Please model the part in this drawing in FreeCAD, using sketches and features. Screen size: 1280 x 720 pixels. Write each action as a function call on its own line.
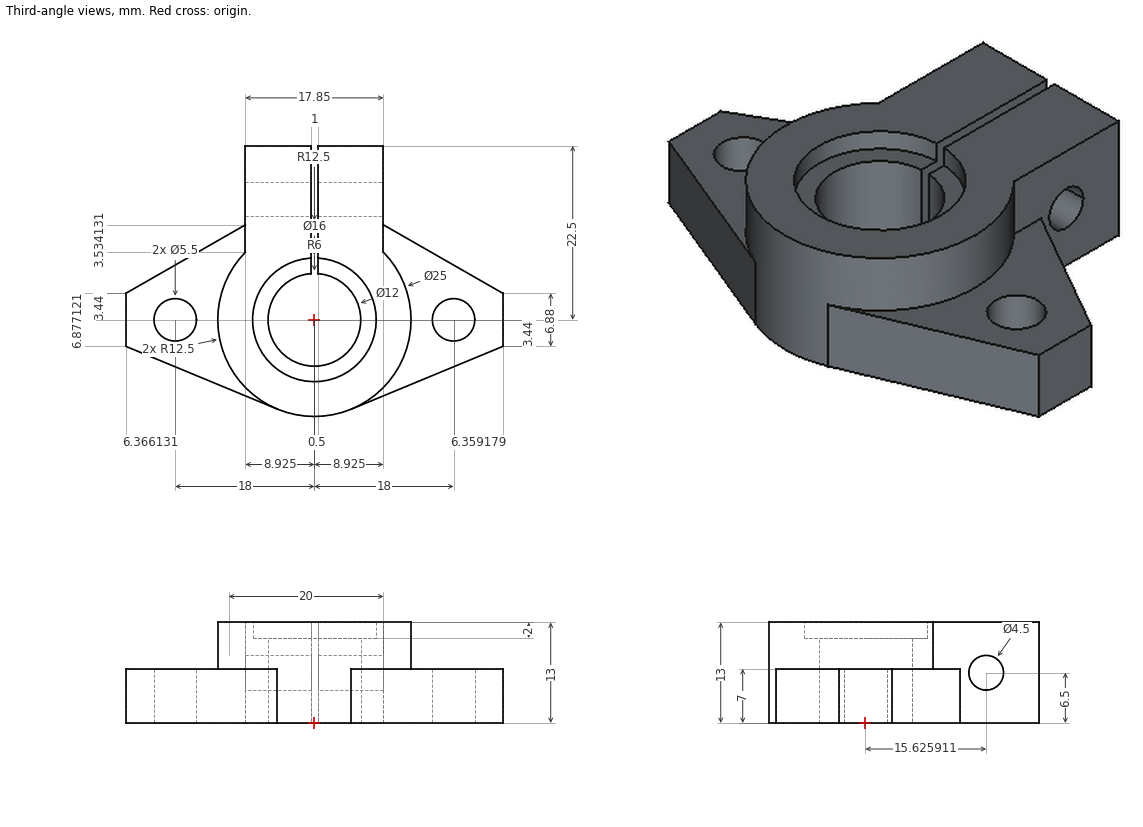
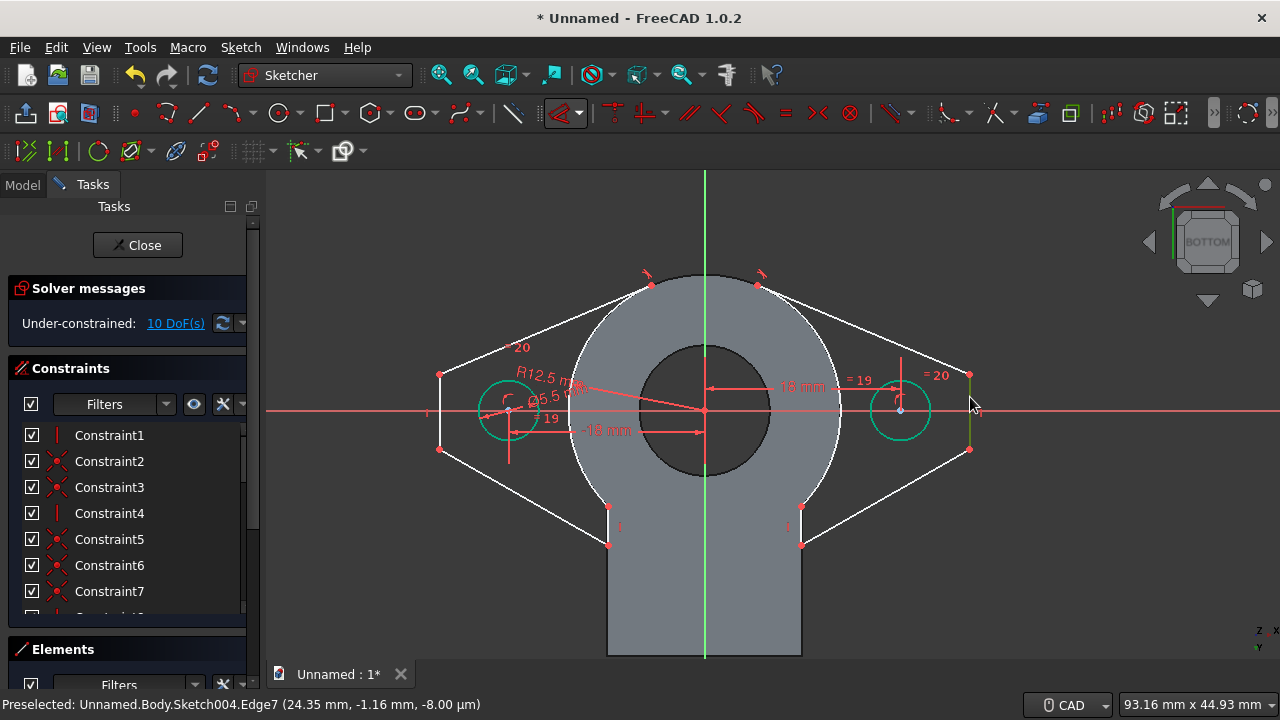
click(582, 114)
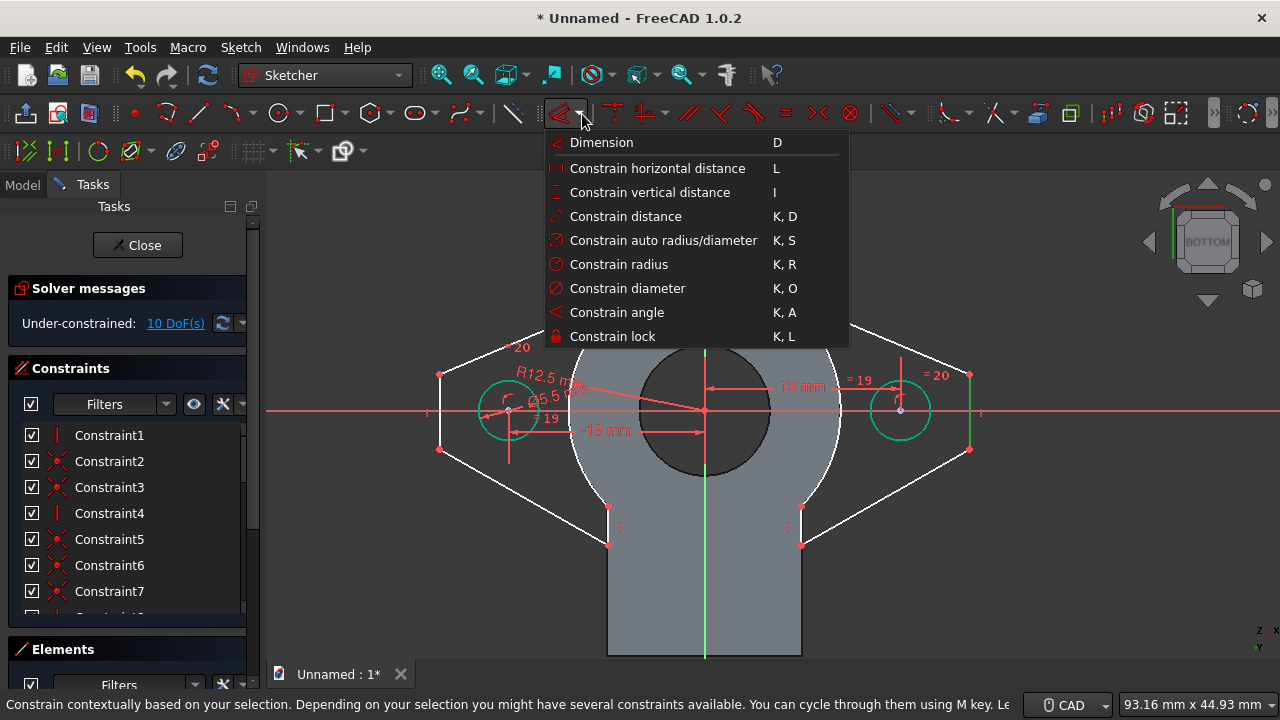
click(697, 192)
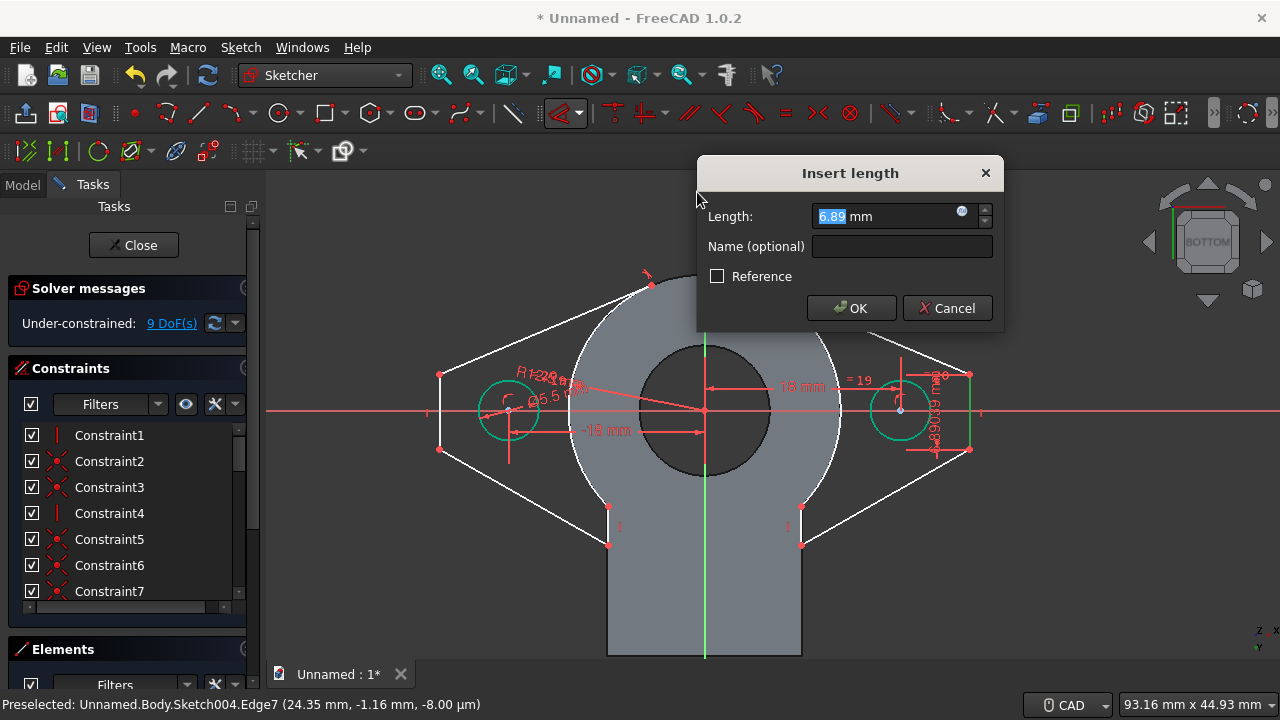
text(6.88)
key(Return)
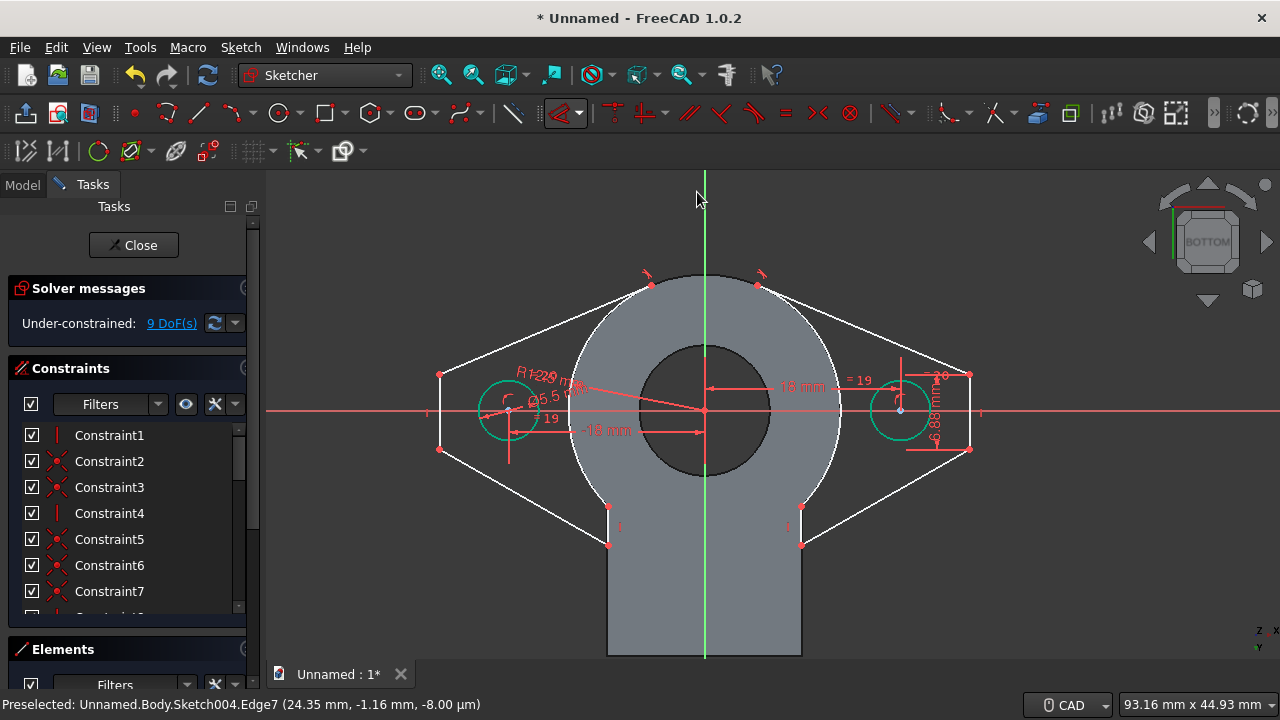
click(440, 450)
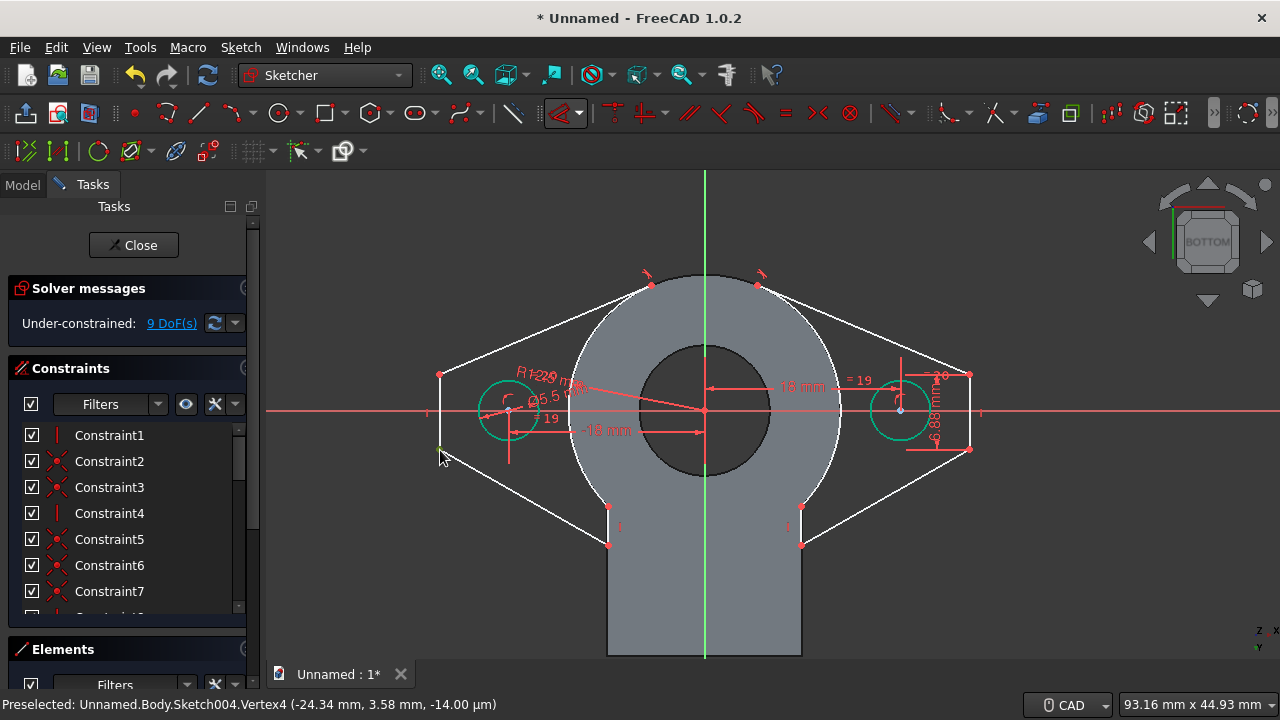
key(i)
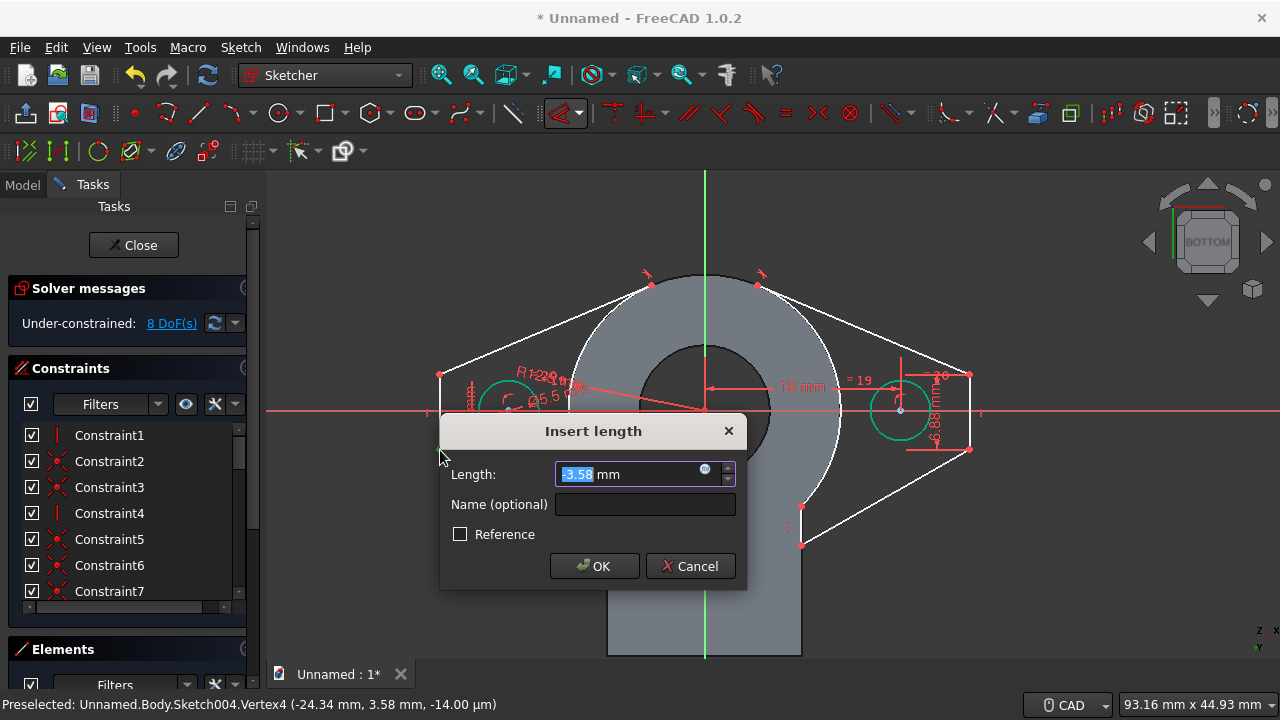
text(-3.44)
key(Return)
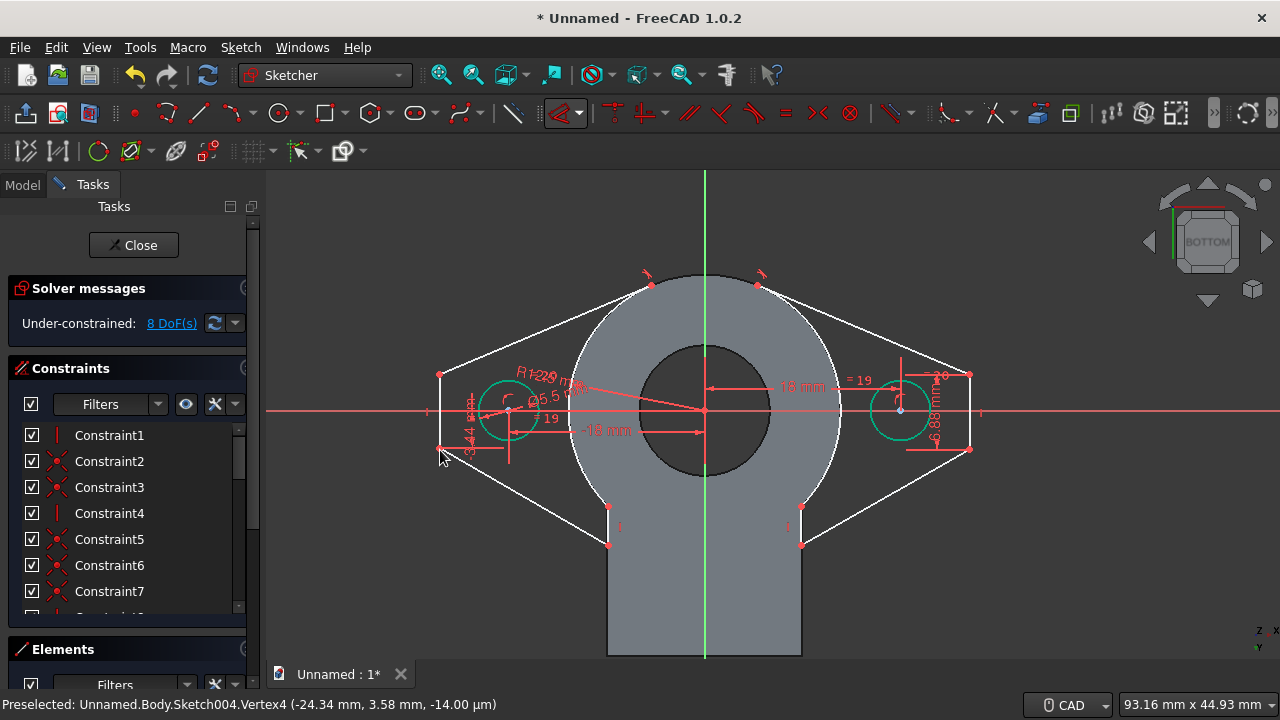
click(970, 375)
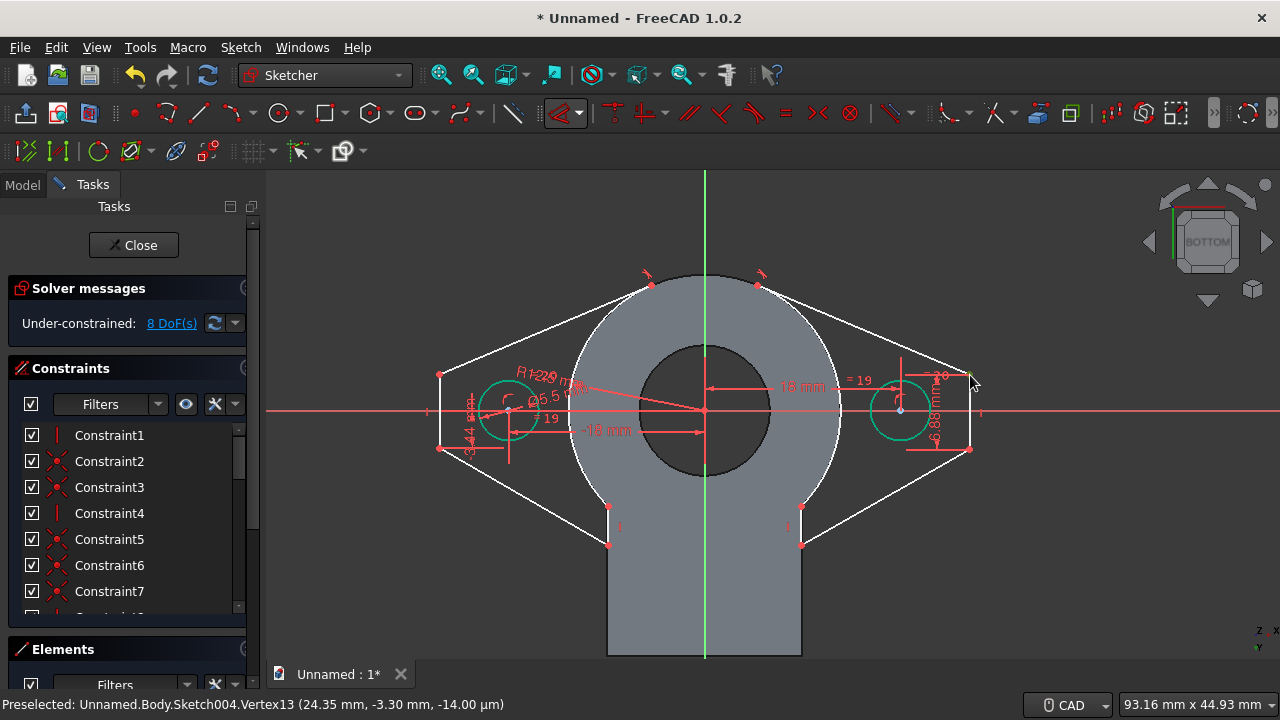
click(582, 114)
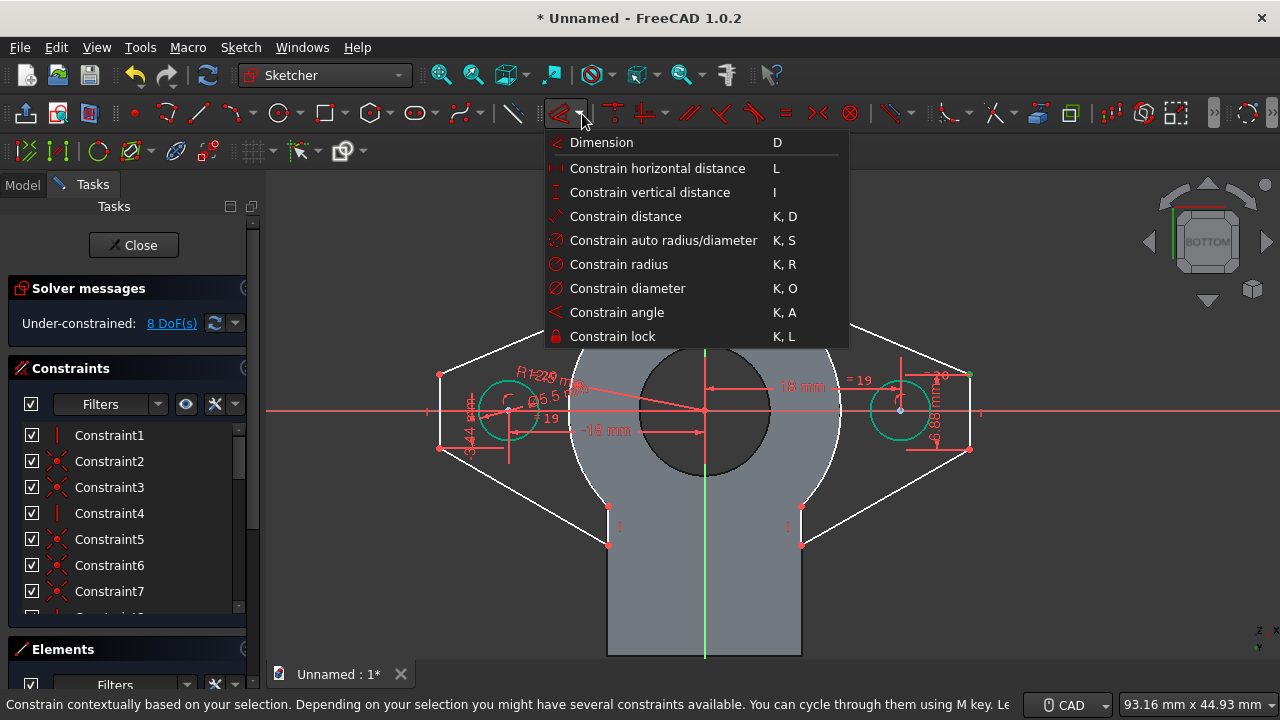
click(697, 192)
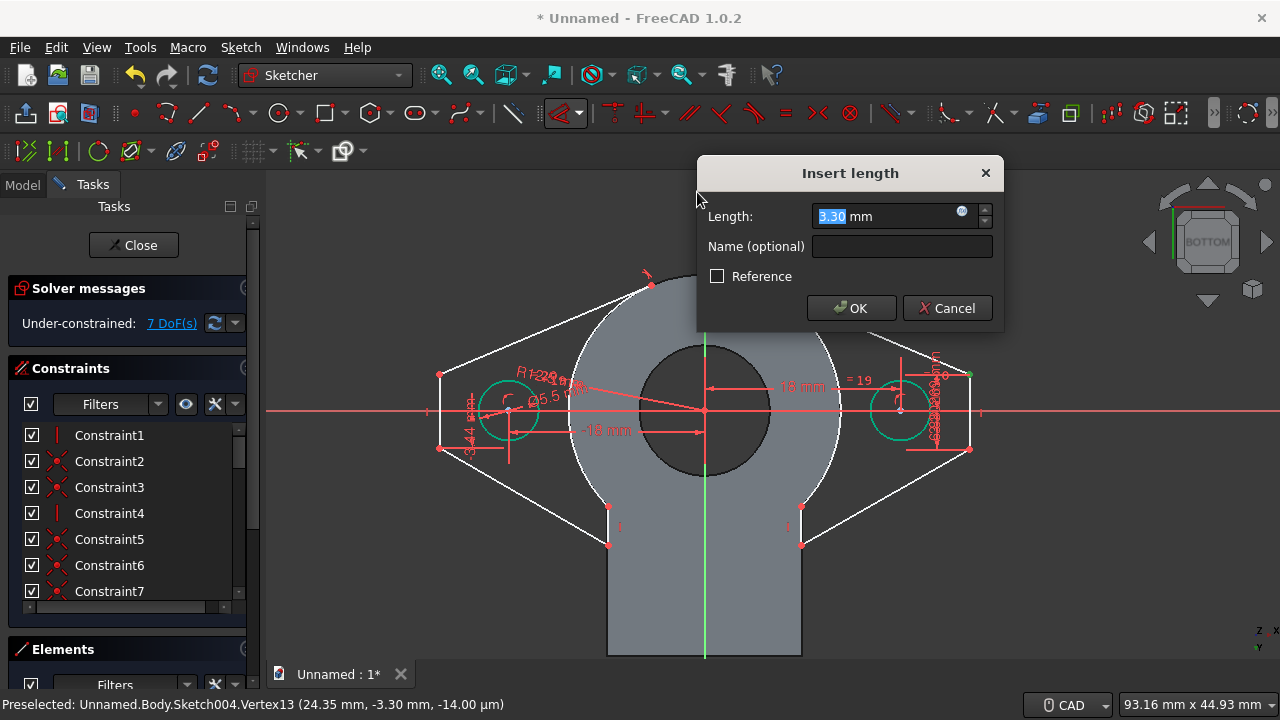
text(3.44)
key(Return)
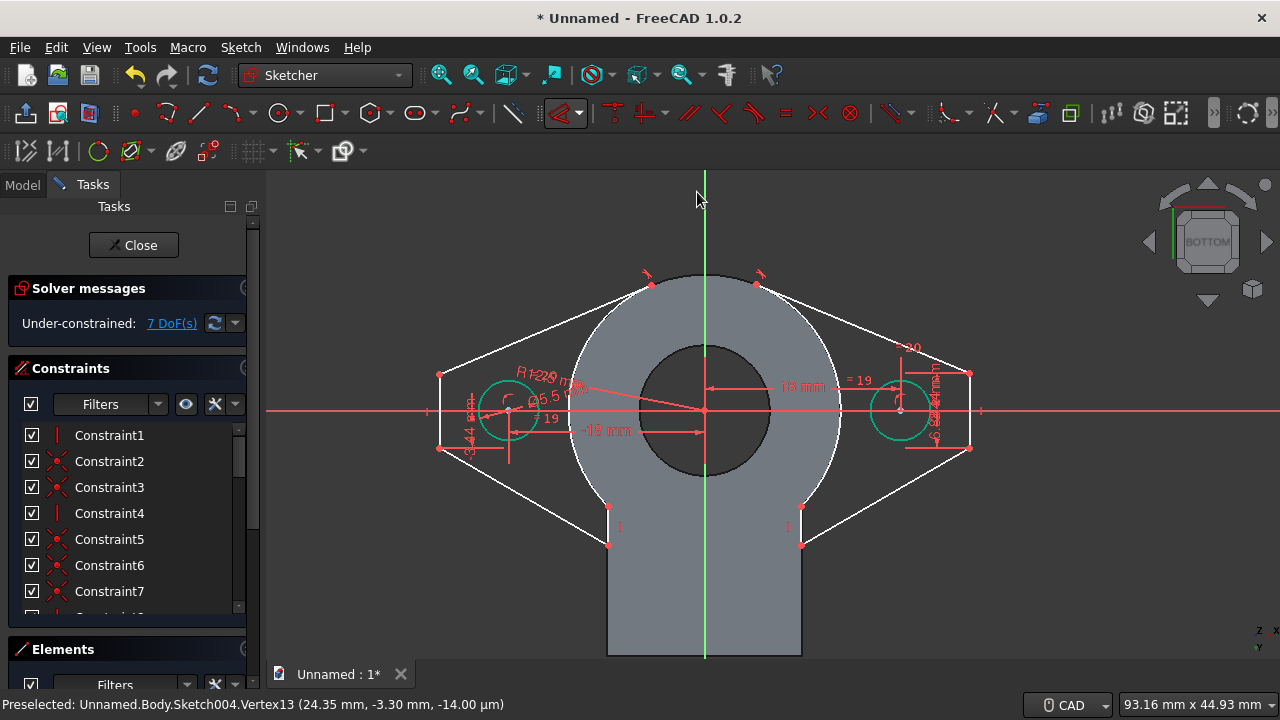
click(608, 507)